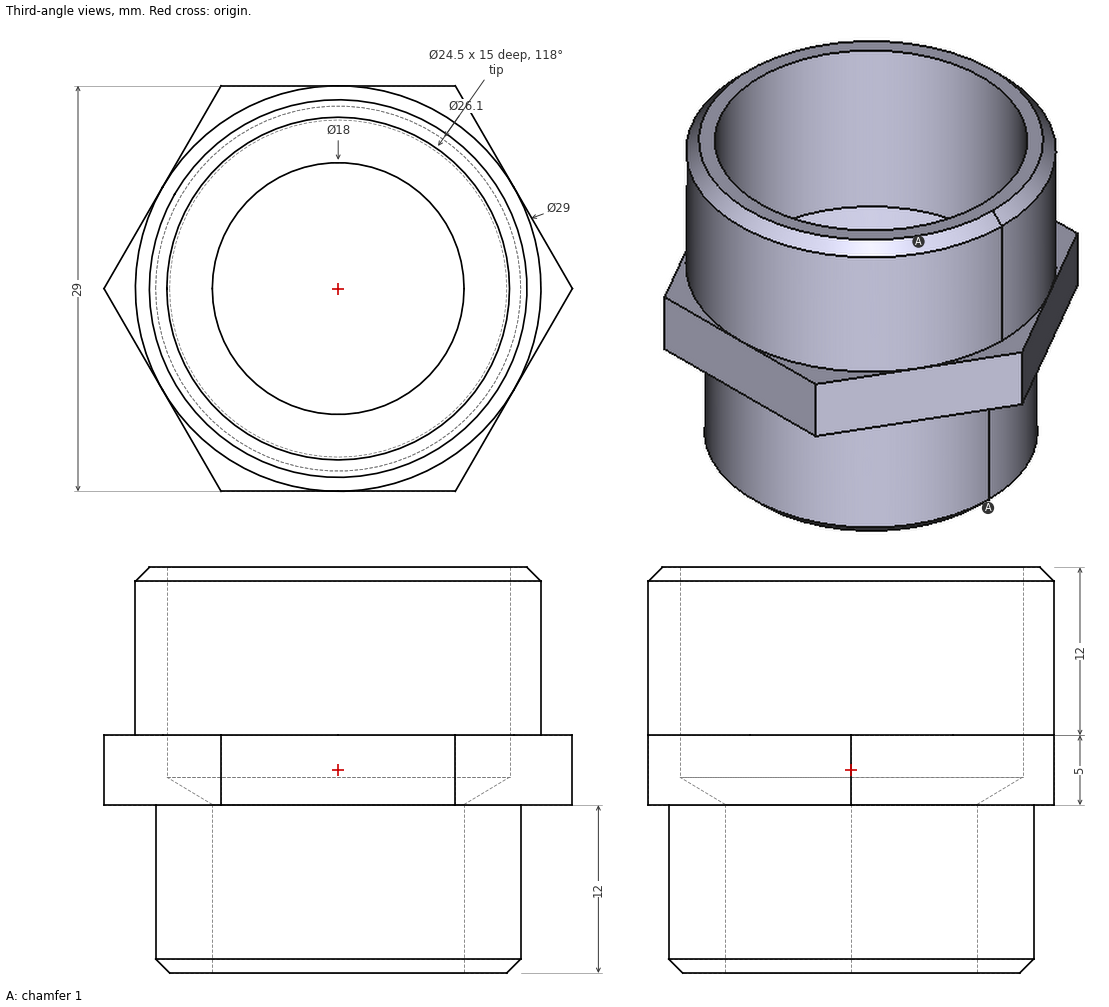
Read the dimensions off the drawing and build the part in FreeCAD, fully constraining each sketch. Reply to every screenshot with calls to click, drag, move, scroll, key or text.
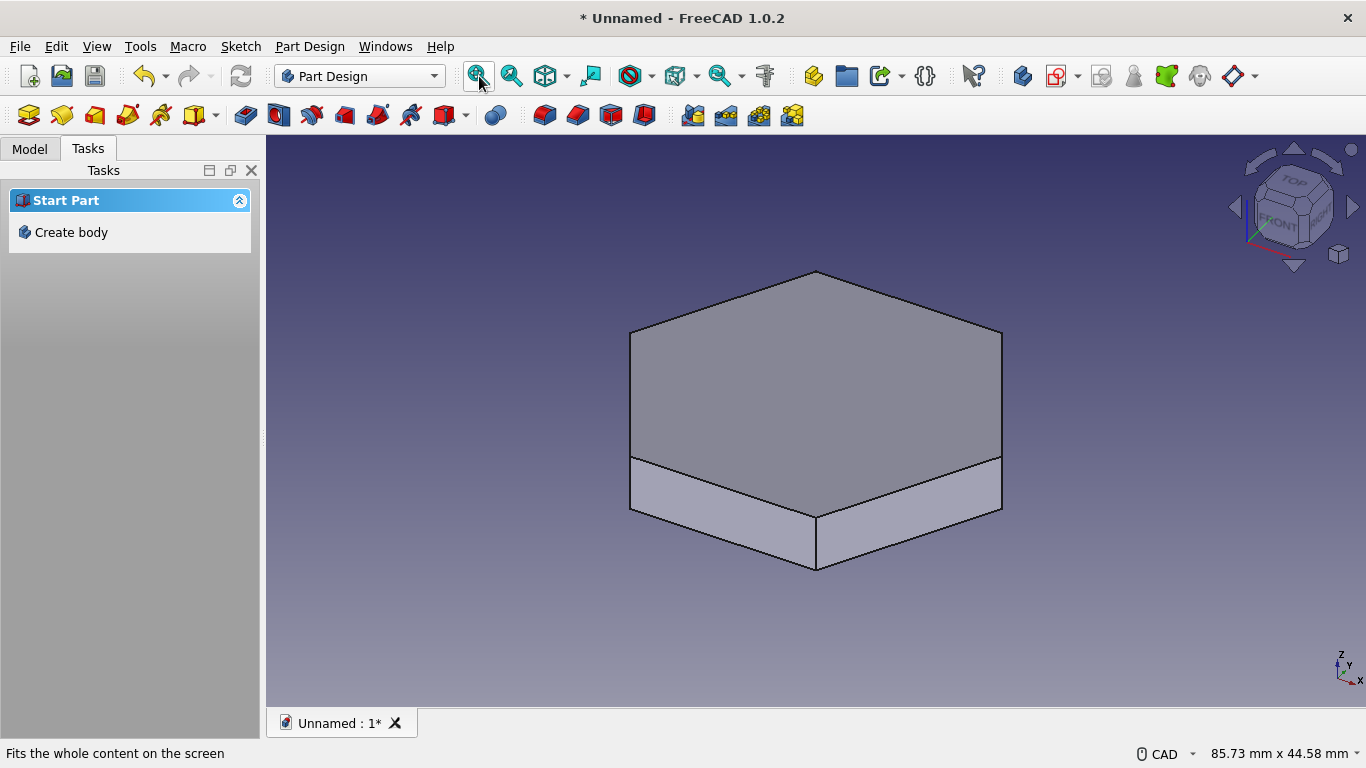
key(5)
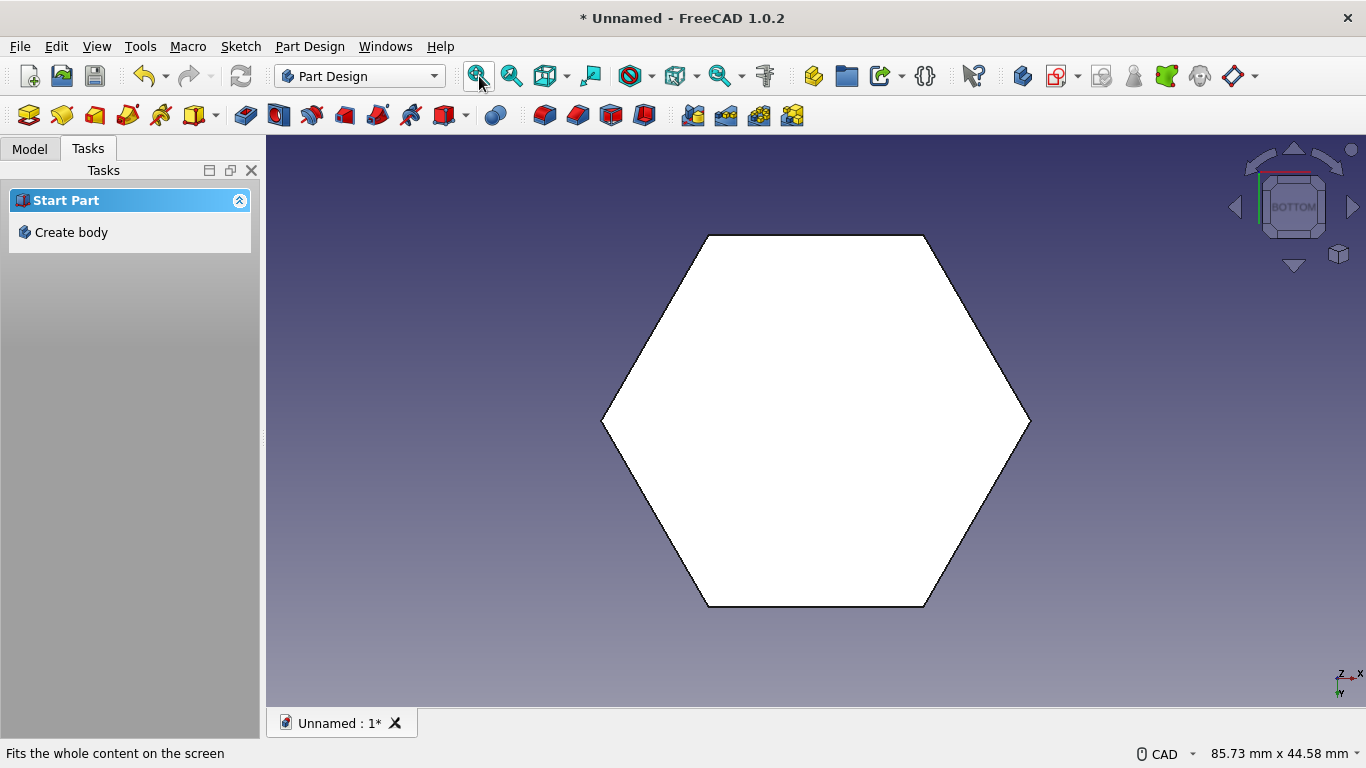
click(816, 420)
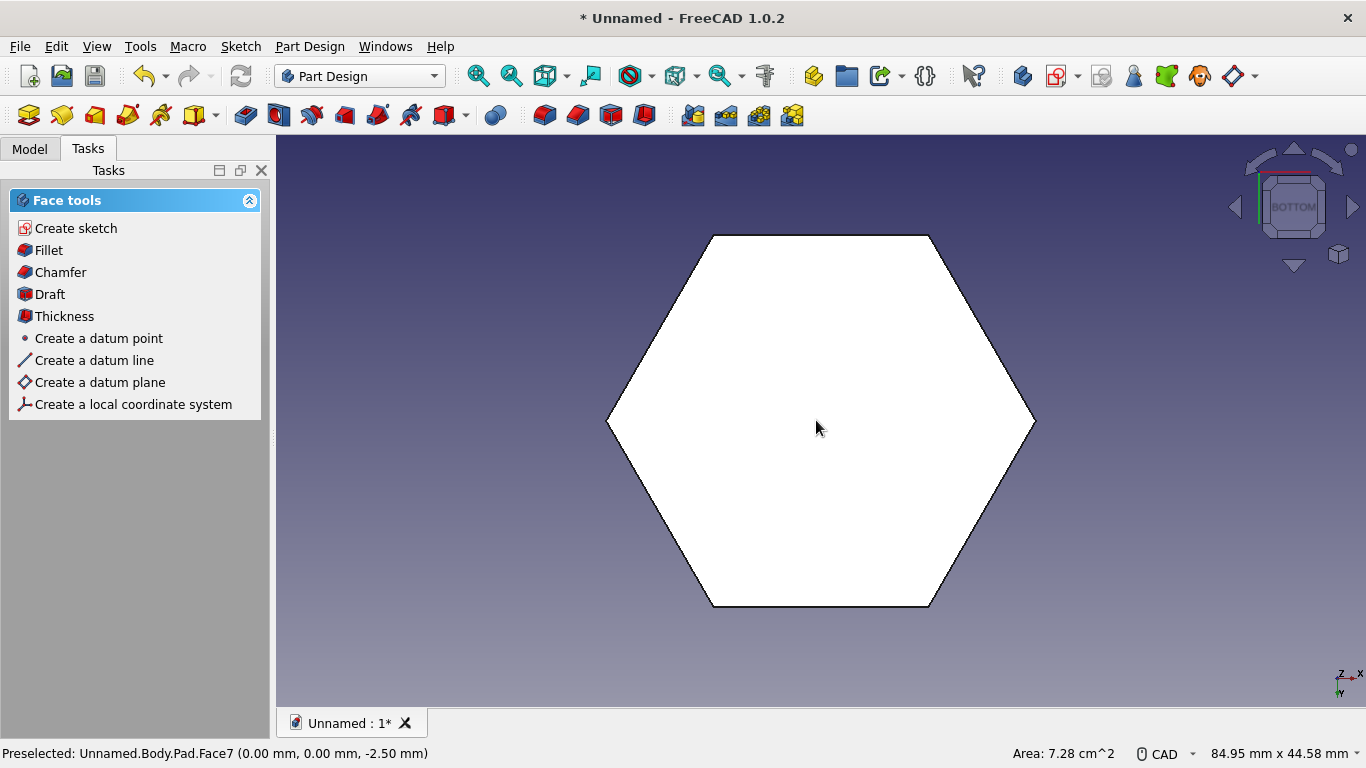
click(1056, 76)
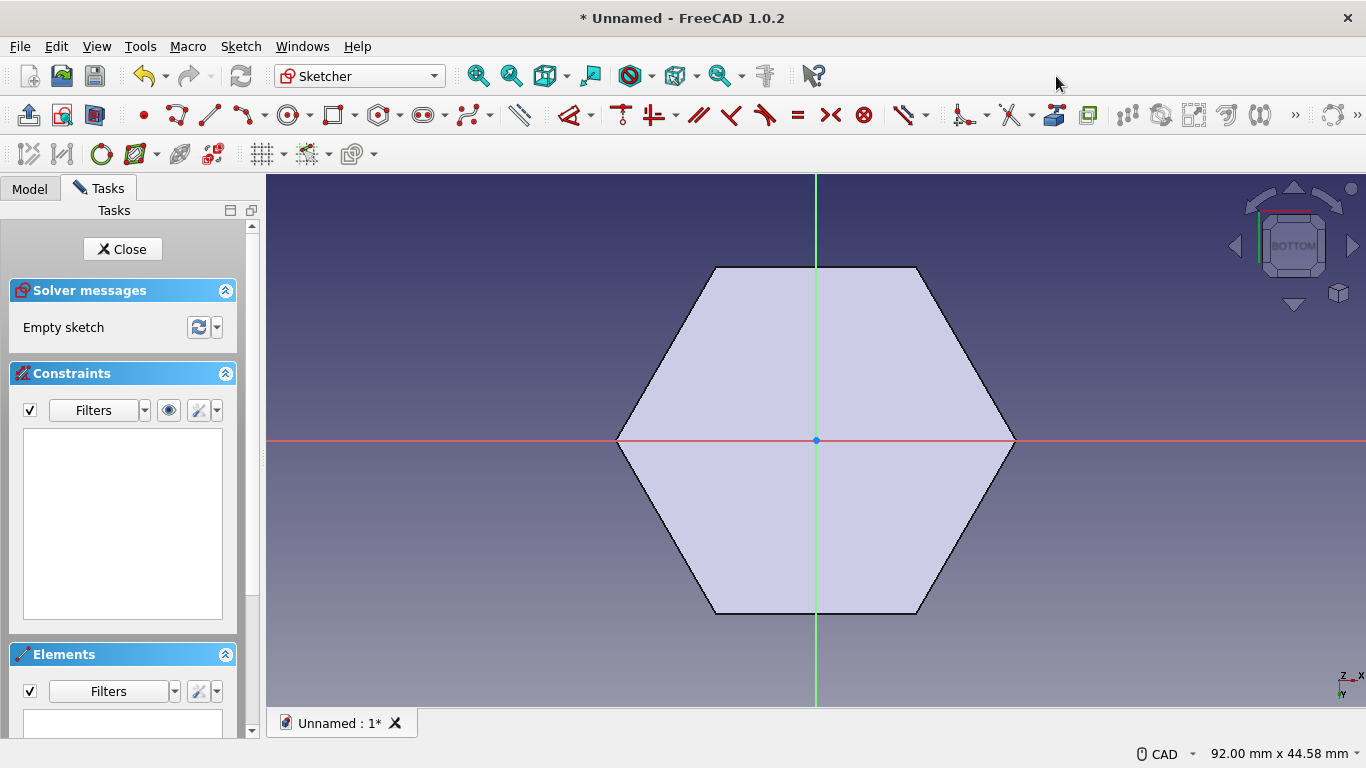
click(288, 116)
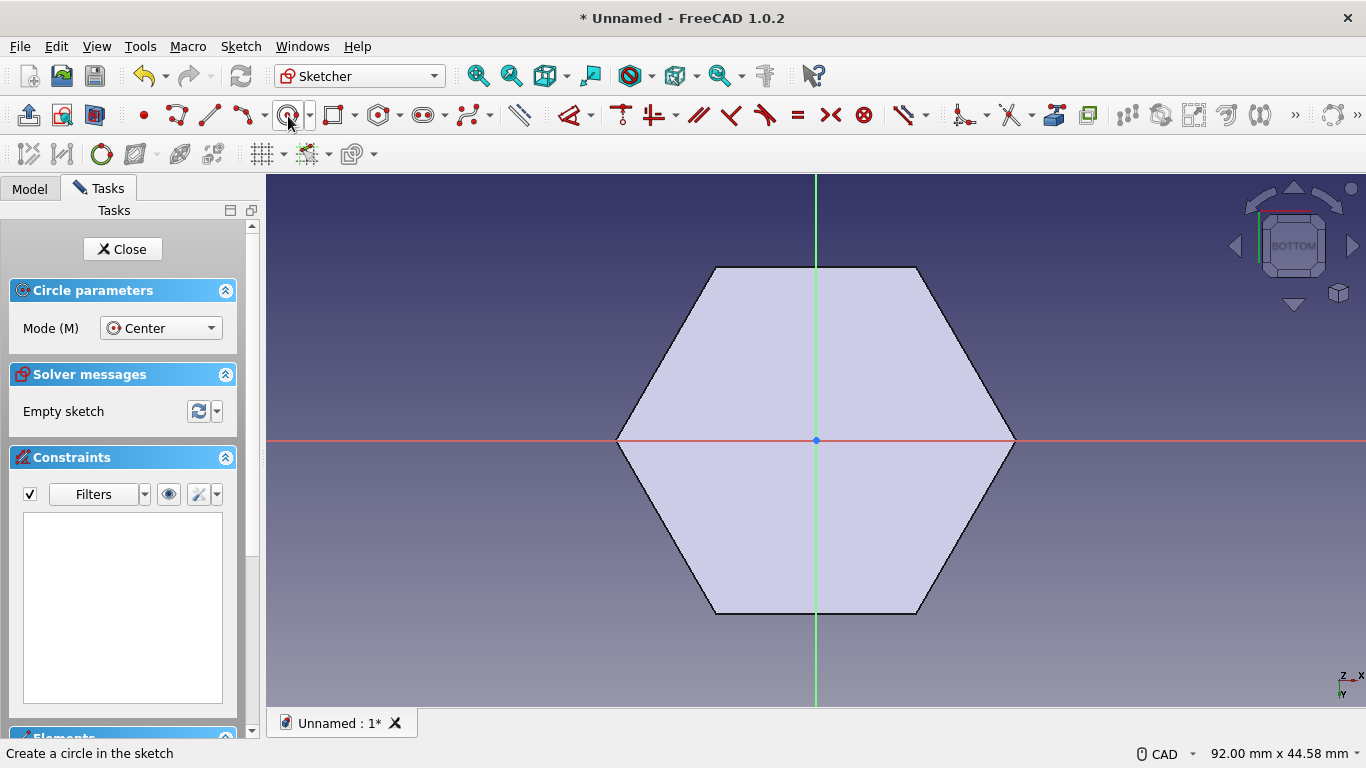
click(816, 440)
move(926, 330)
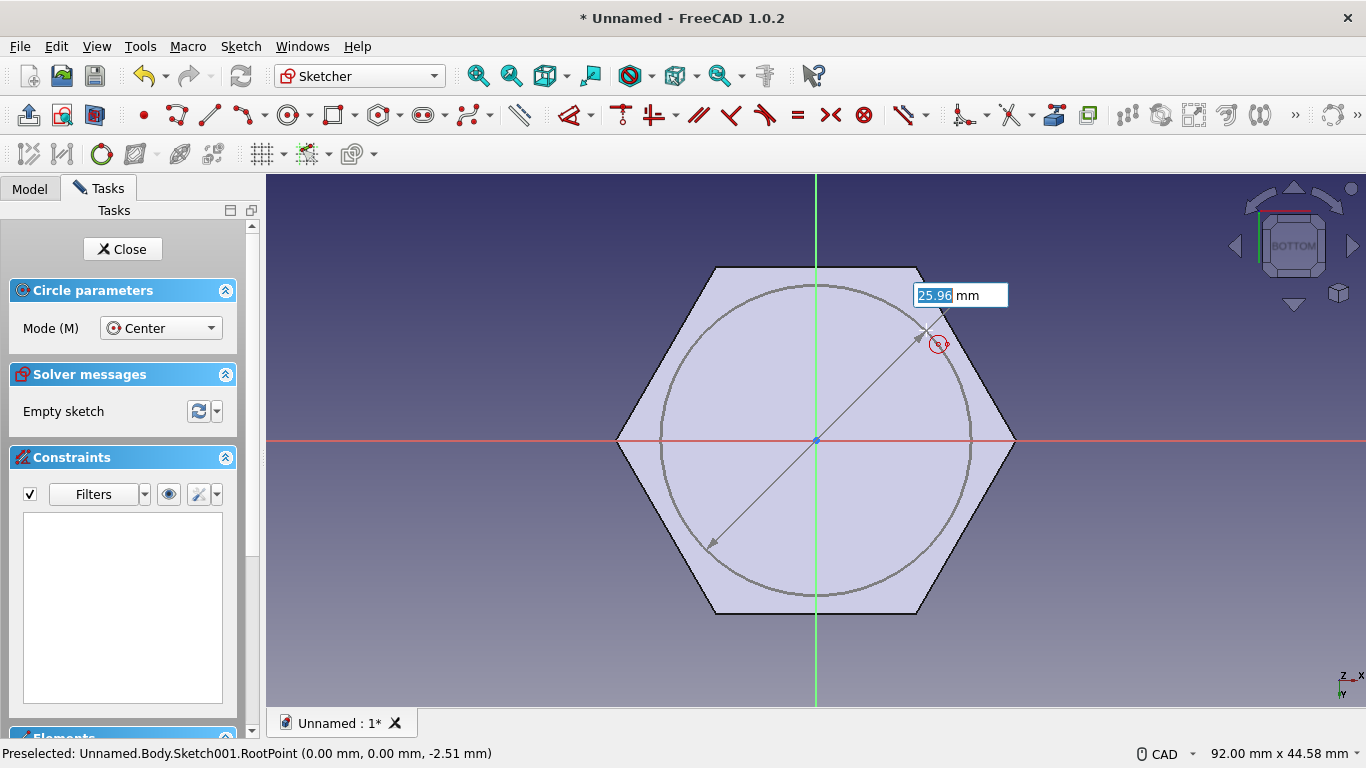
text(26.1)
key(Return)
key(Escape)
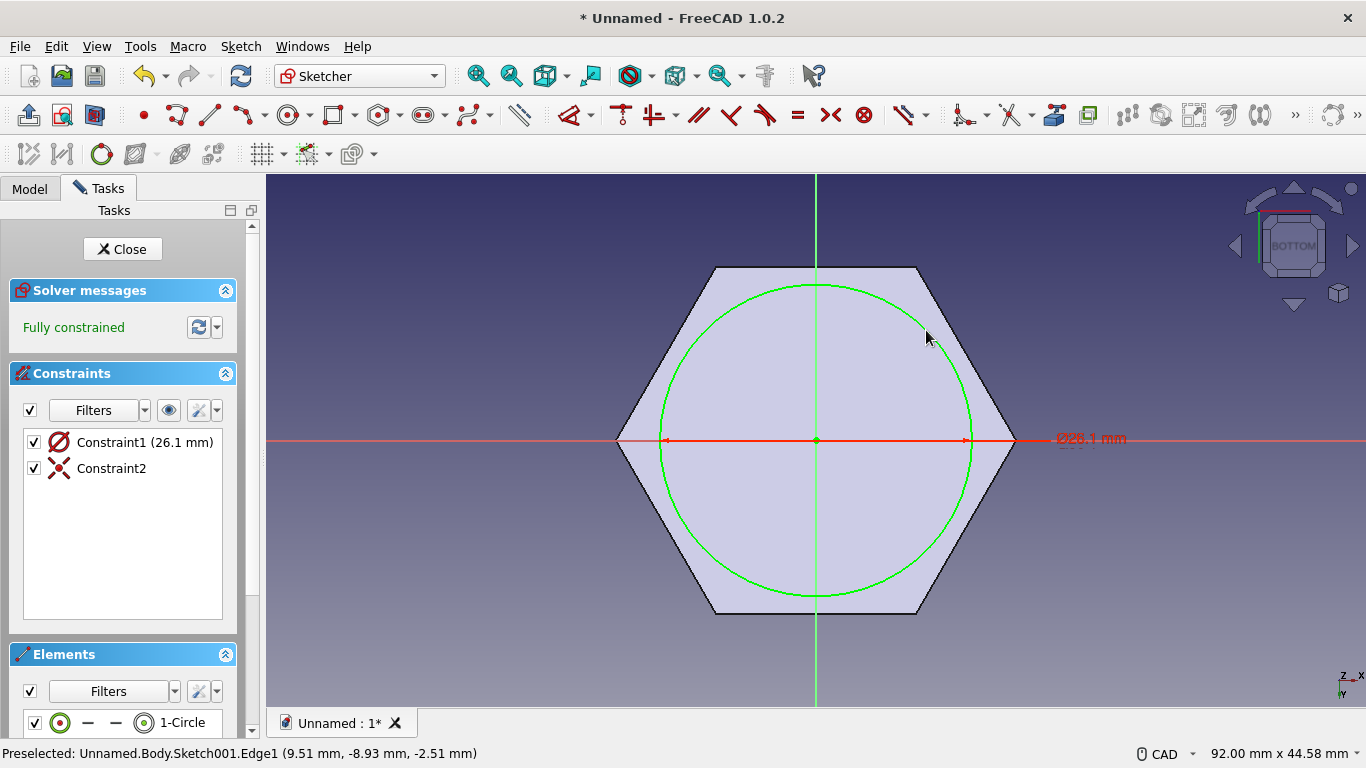
click(123, 249)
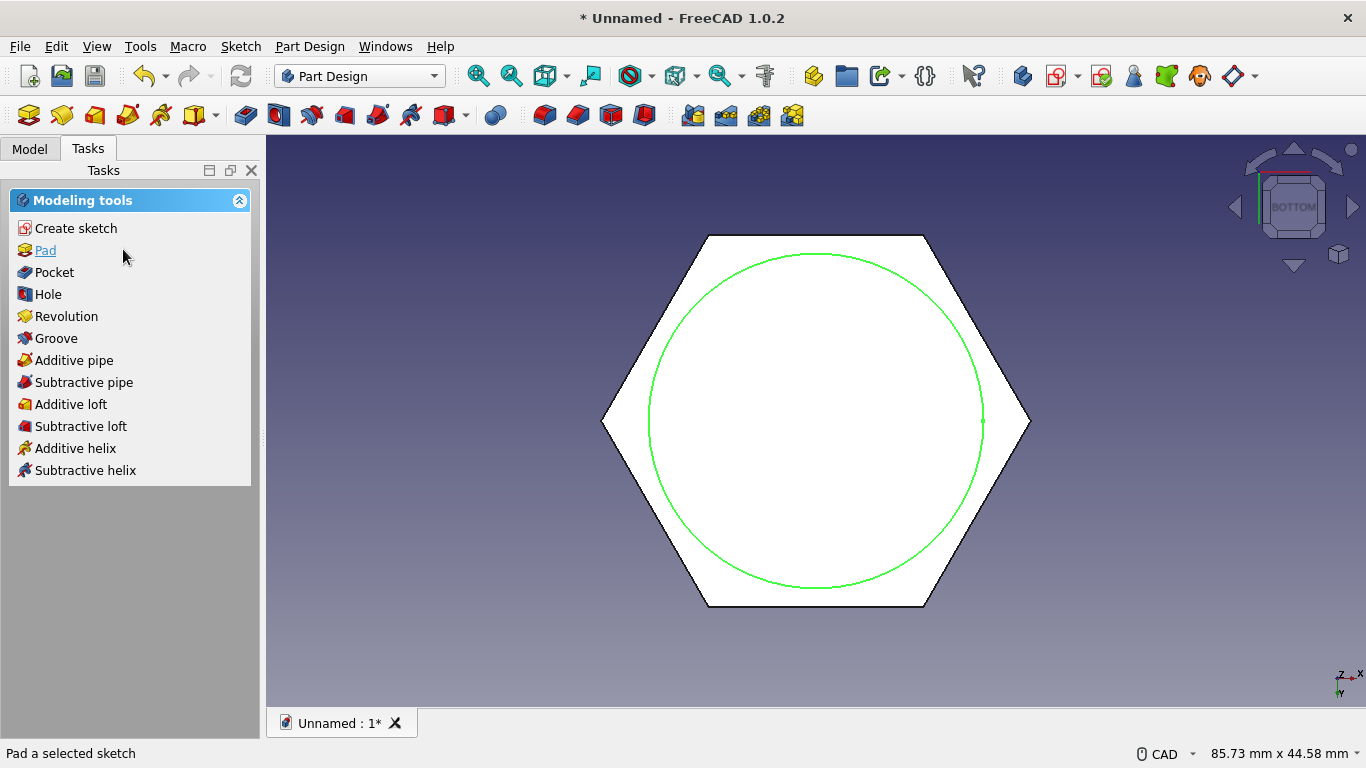
click(29, 116)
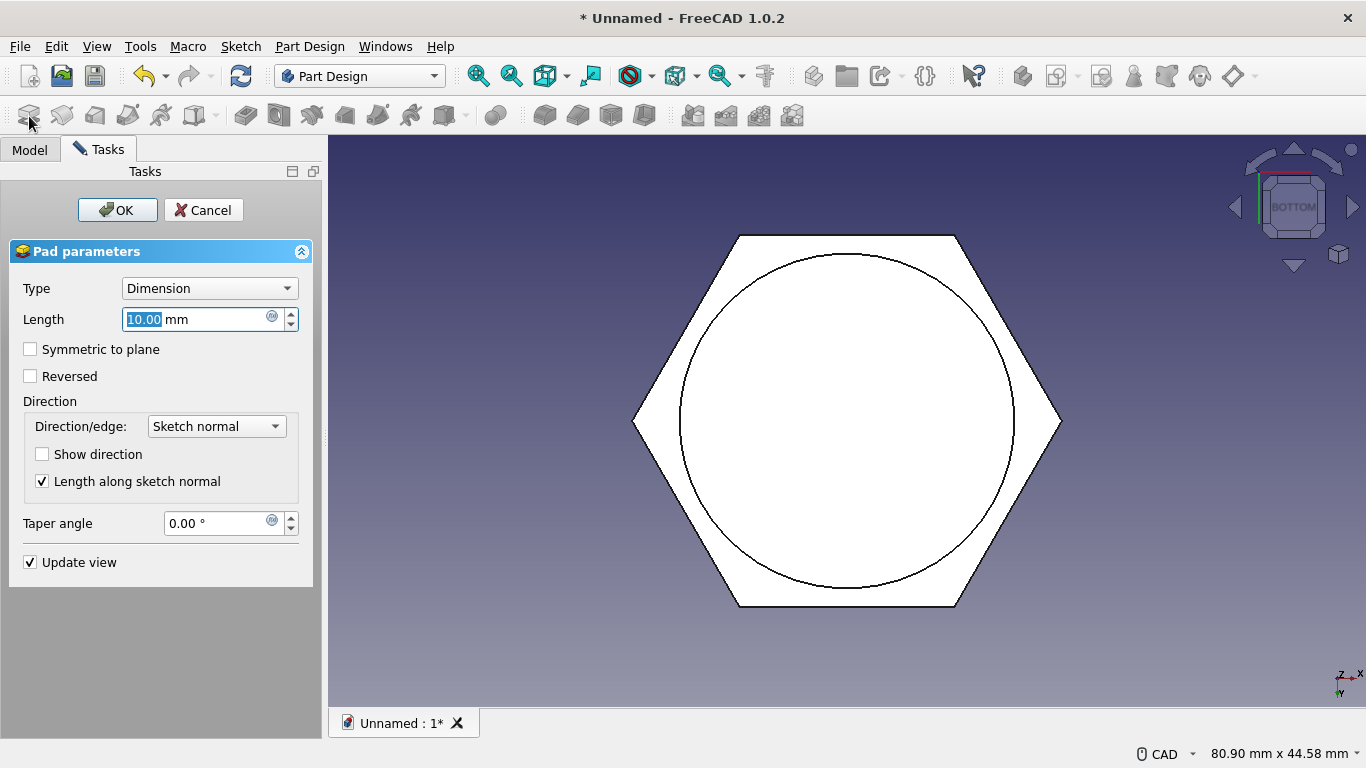
text(12)
key(Tab)